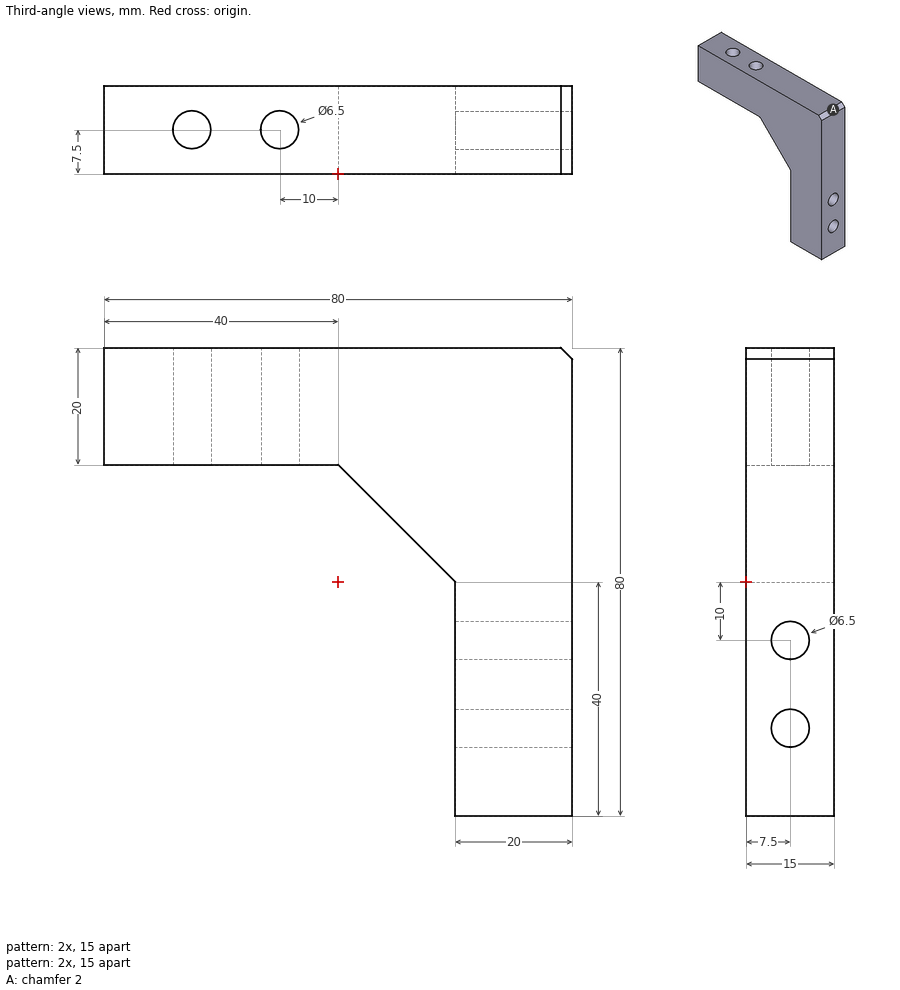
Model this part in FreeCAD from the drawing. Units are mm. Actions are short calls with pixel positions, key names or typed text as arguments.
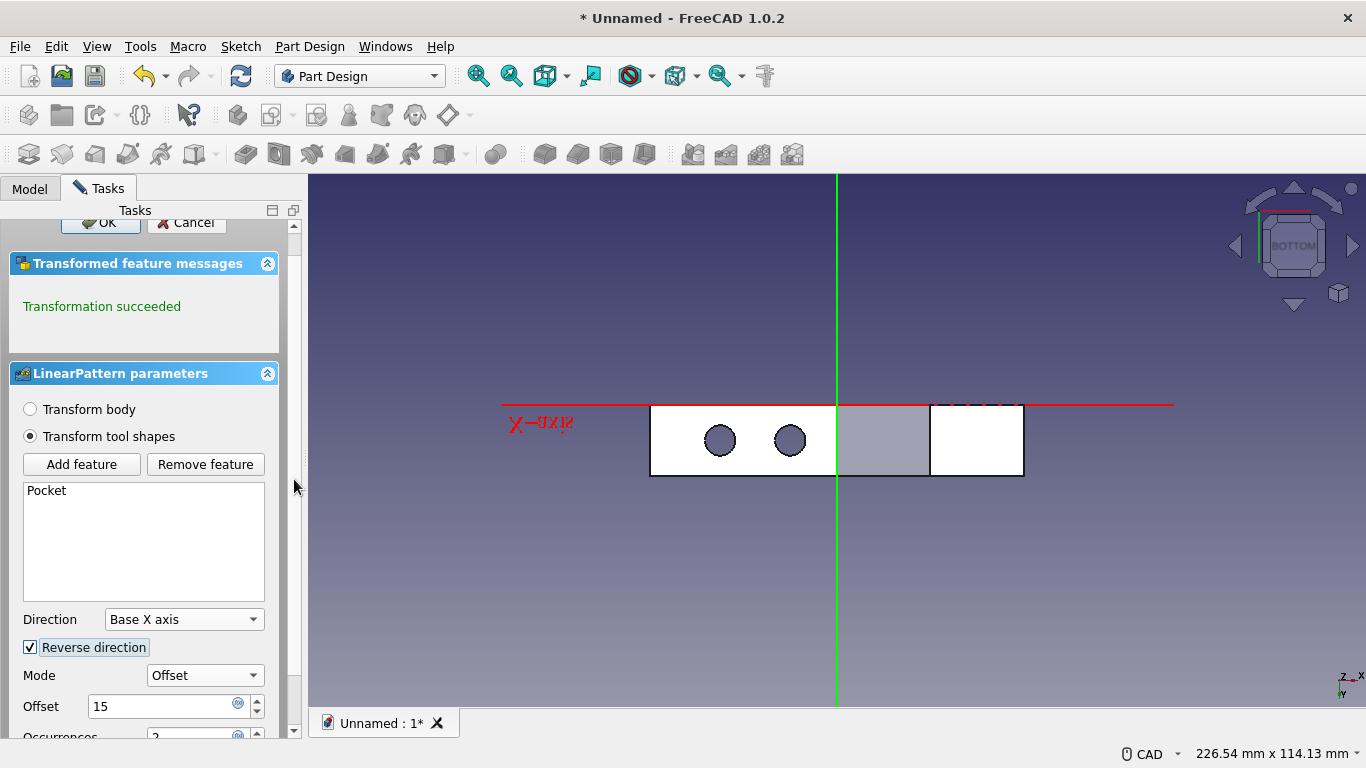
click(101, 249)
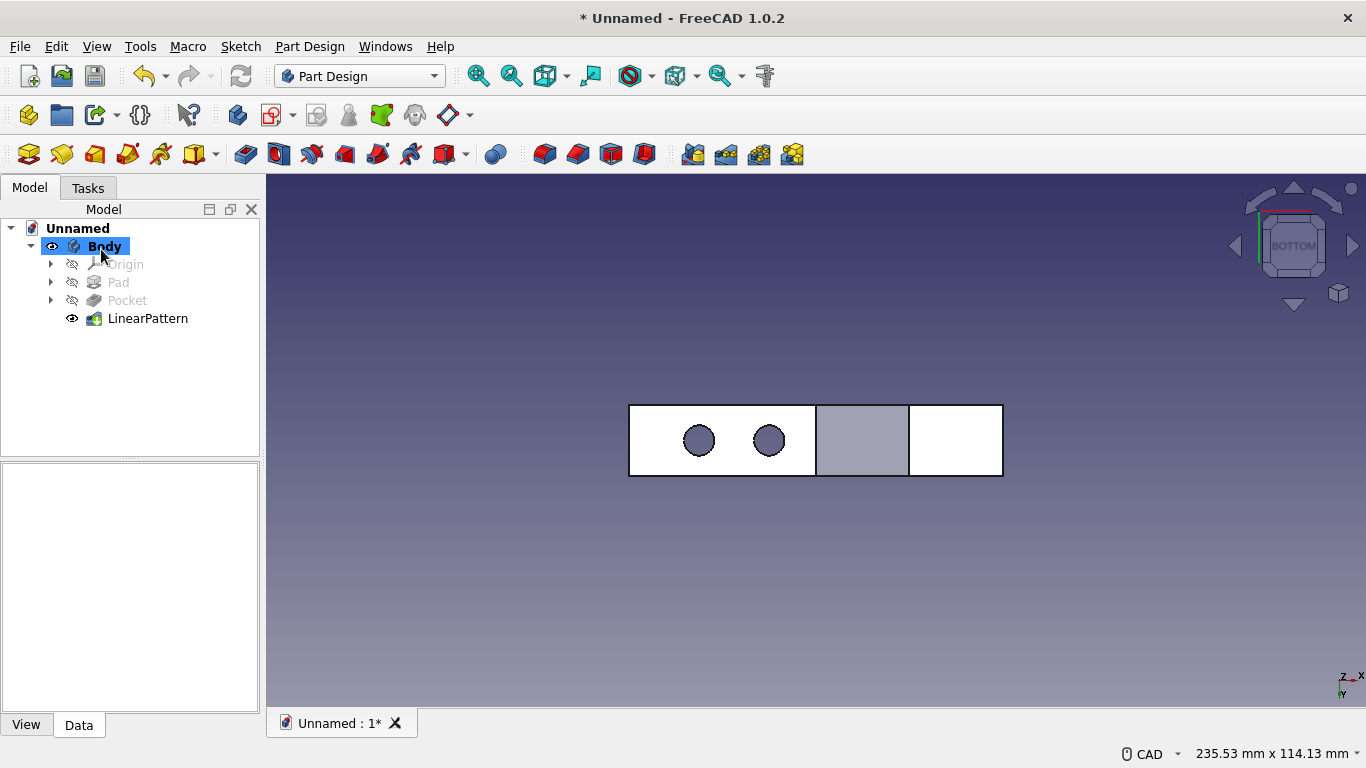
key(v)
key(f)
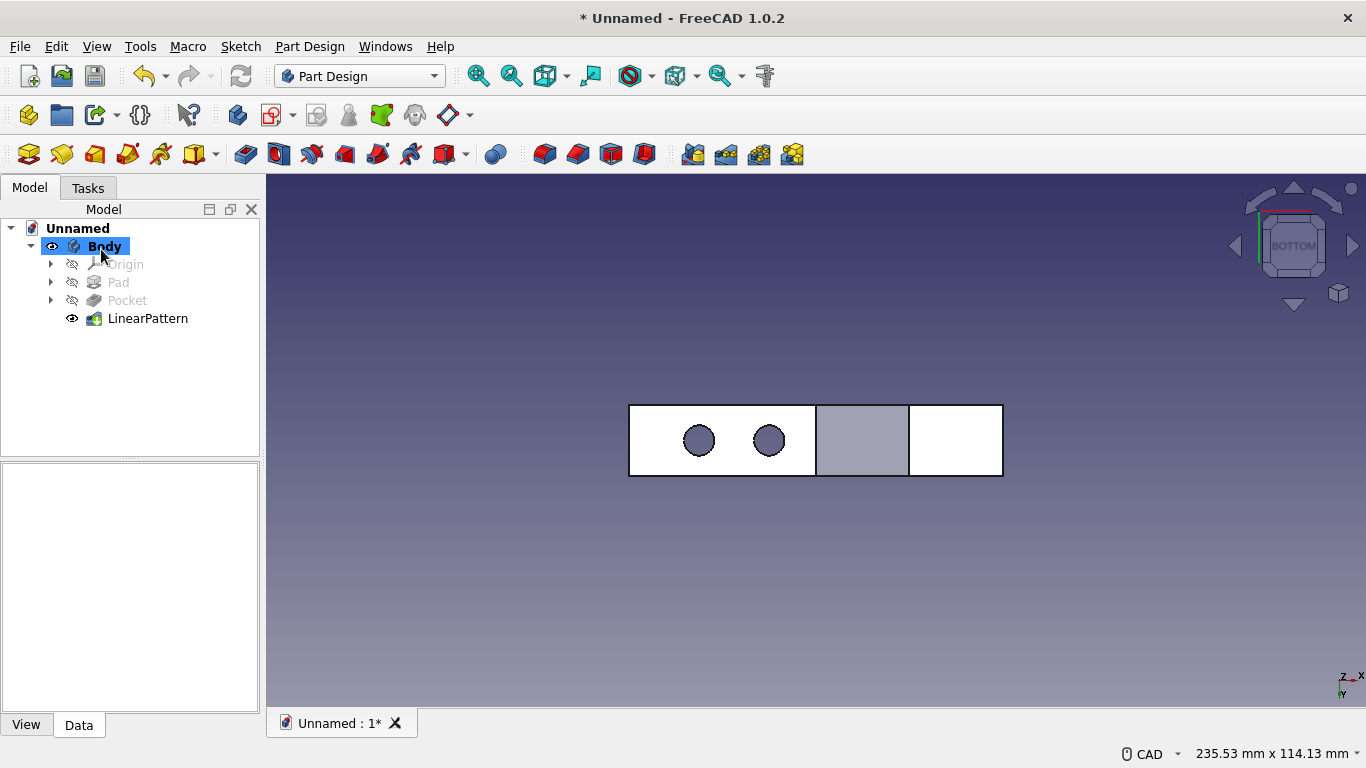
key(0)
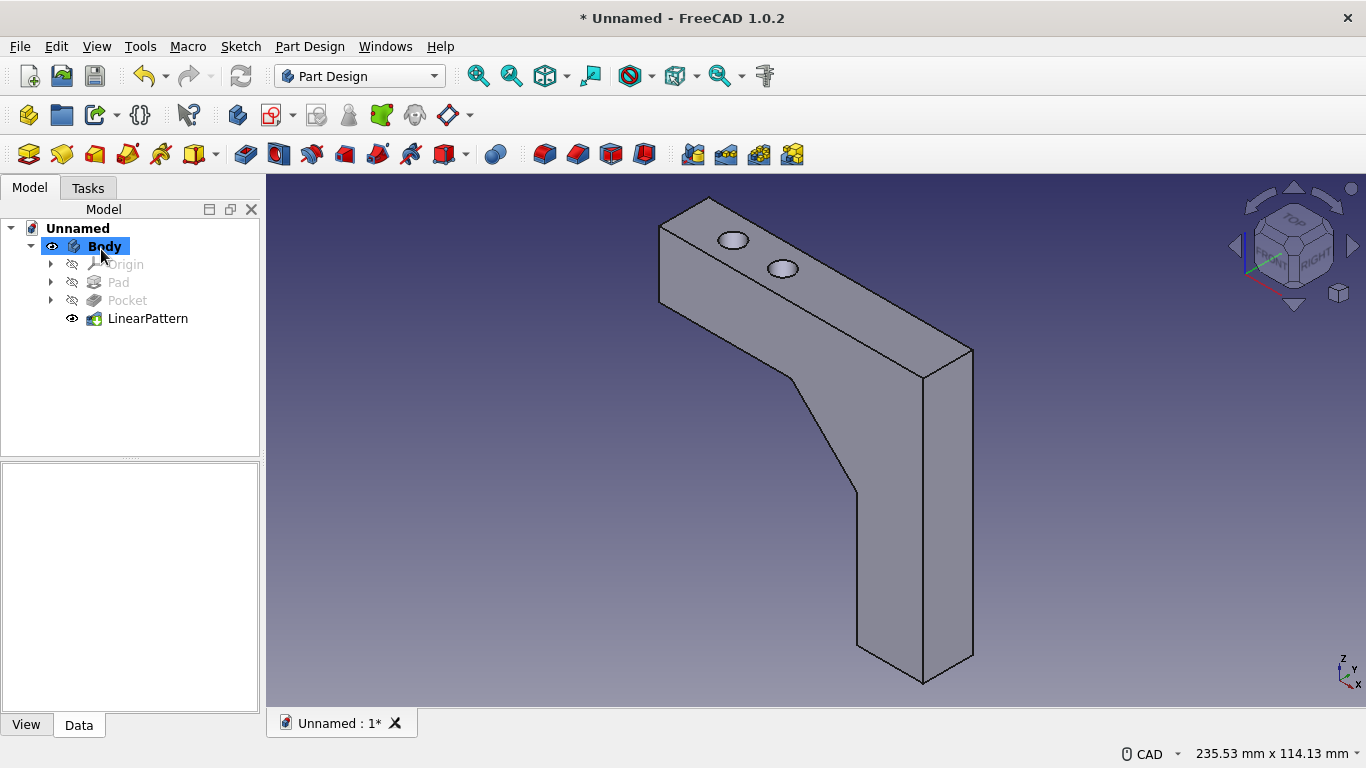
click(948, 516)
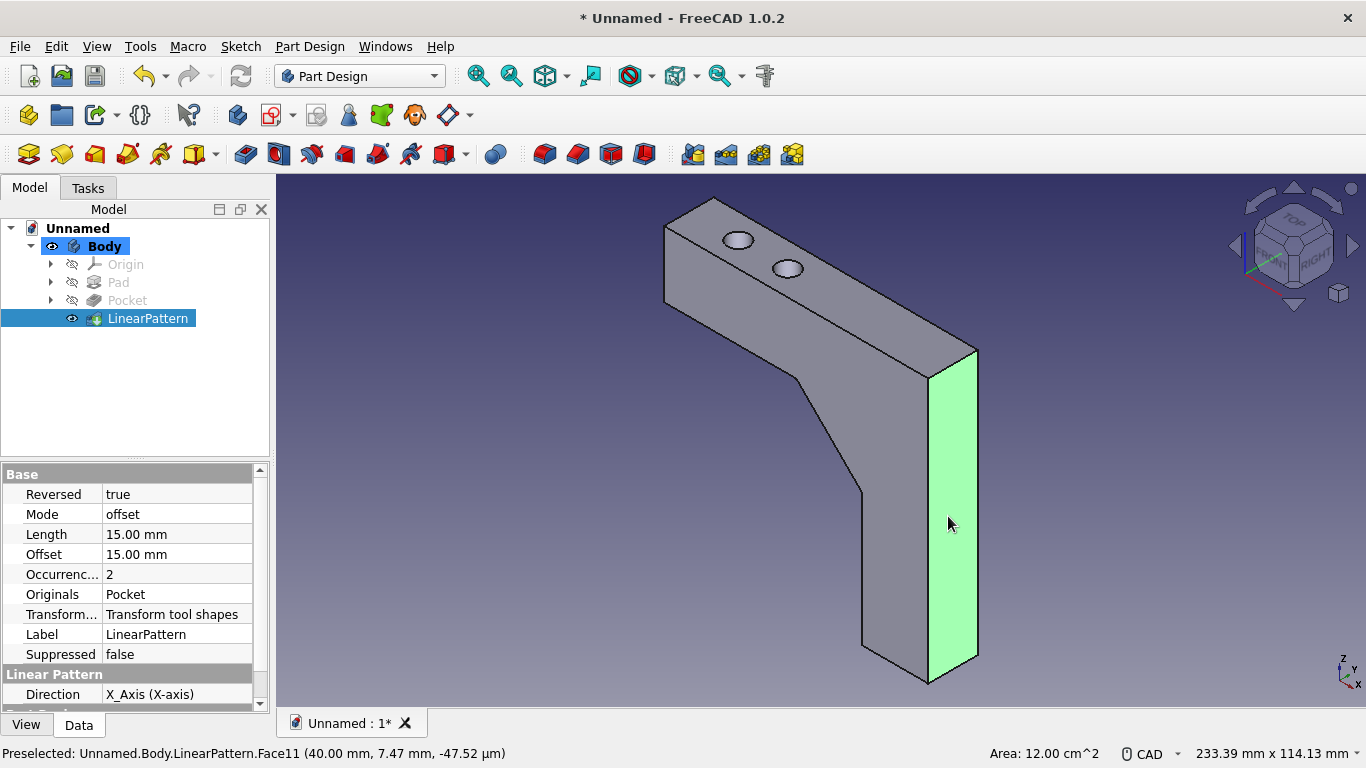
click(270, 116)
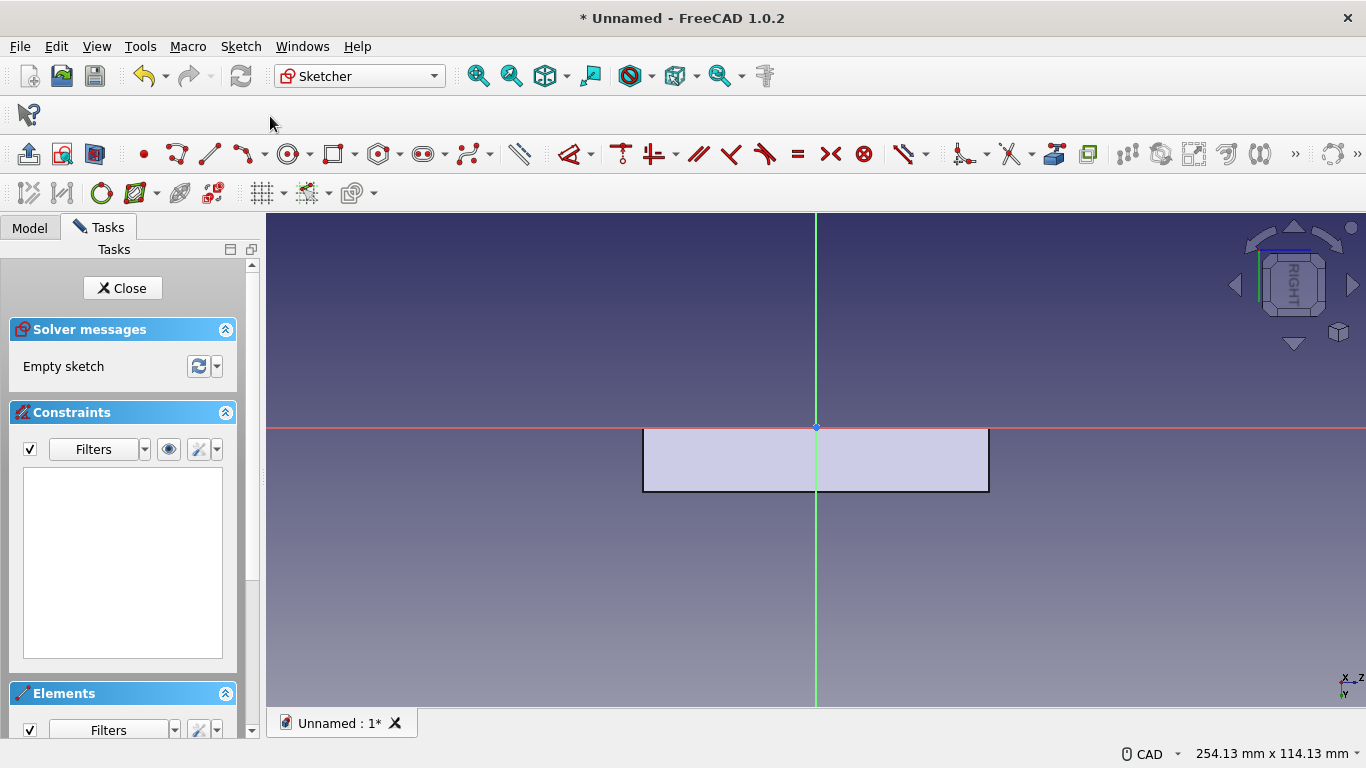
scroll(795, 449, up, 9)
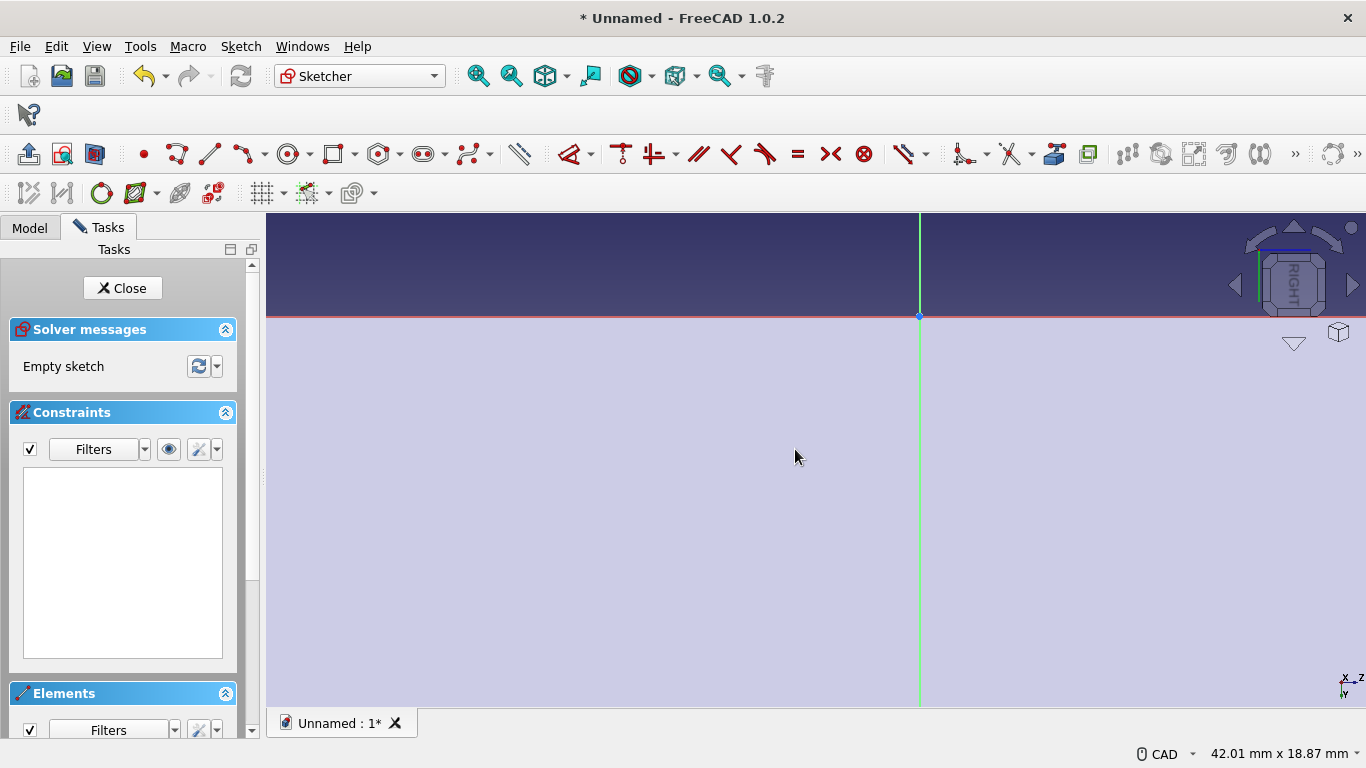
key(g)
key(c)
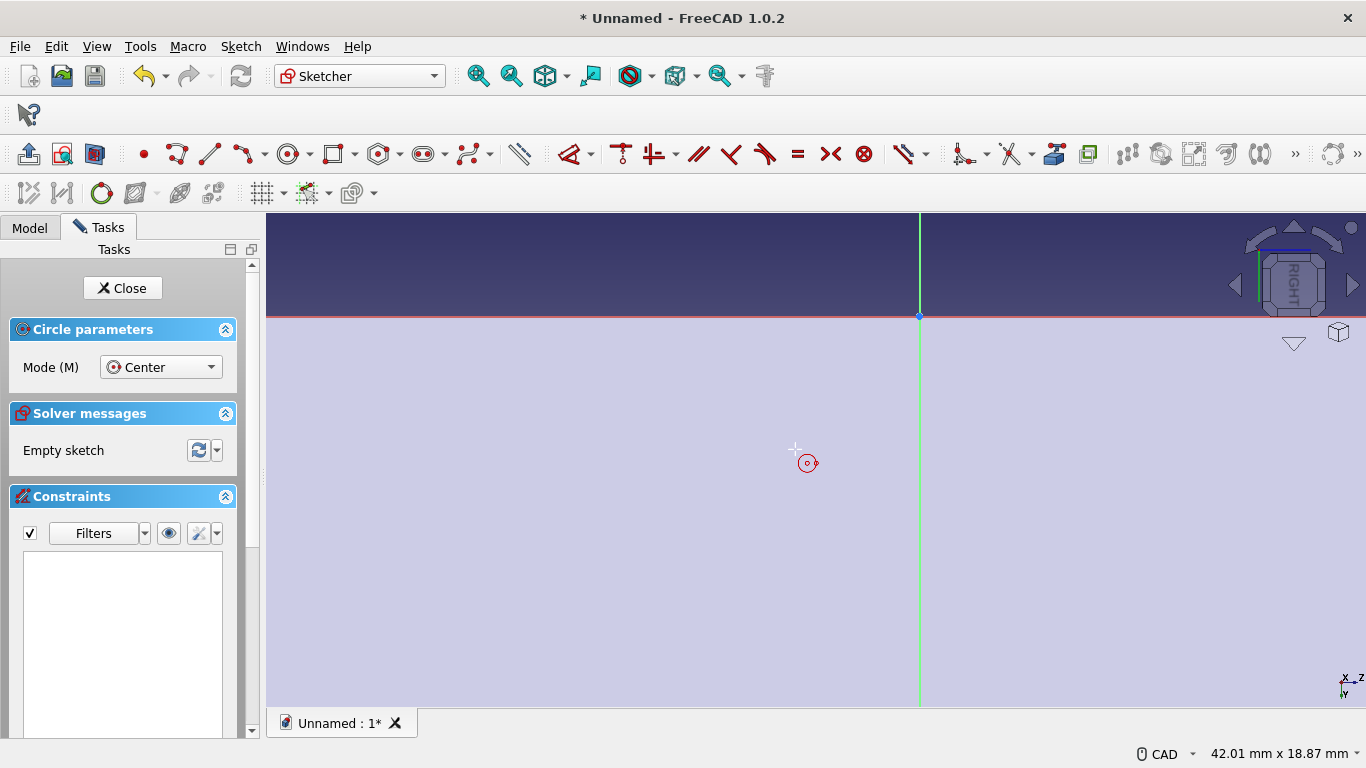
click(658, 513)
move(718, 453)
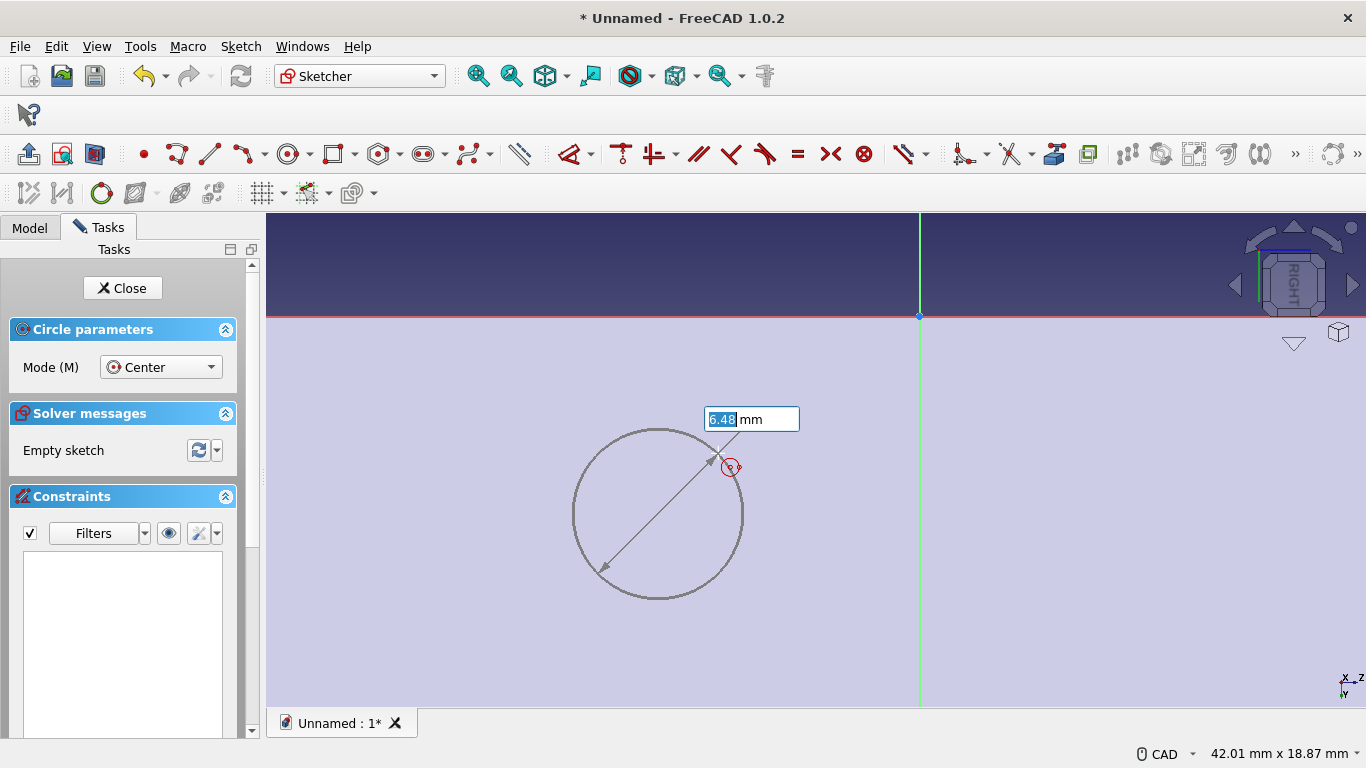
text(6.5)
key(Return)
key(Escape)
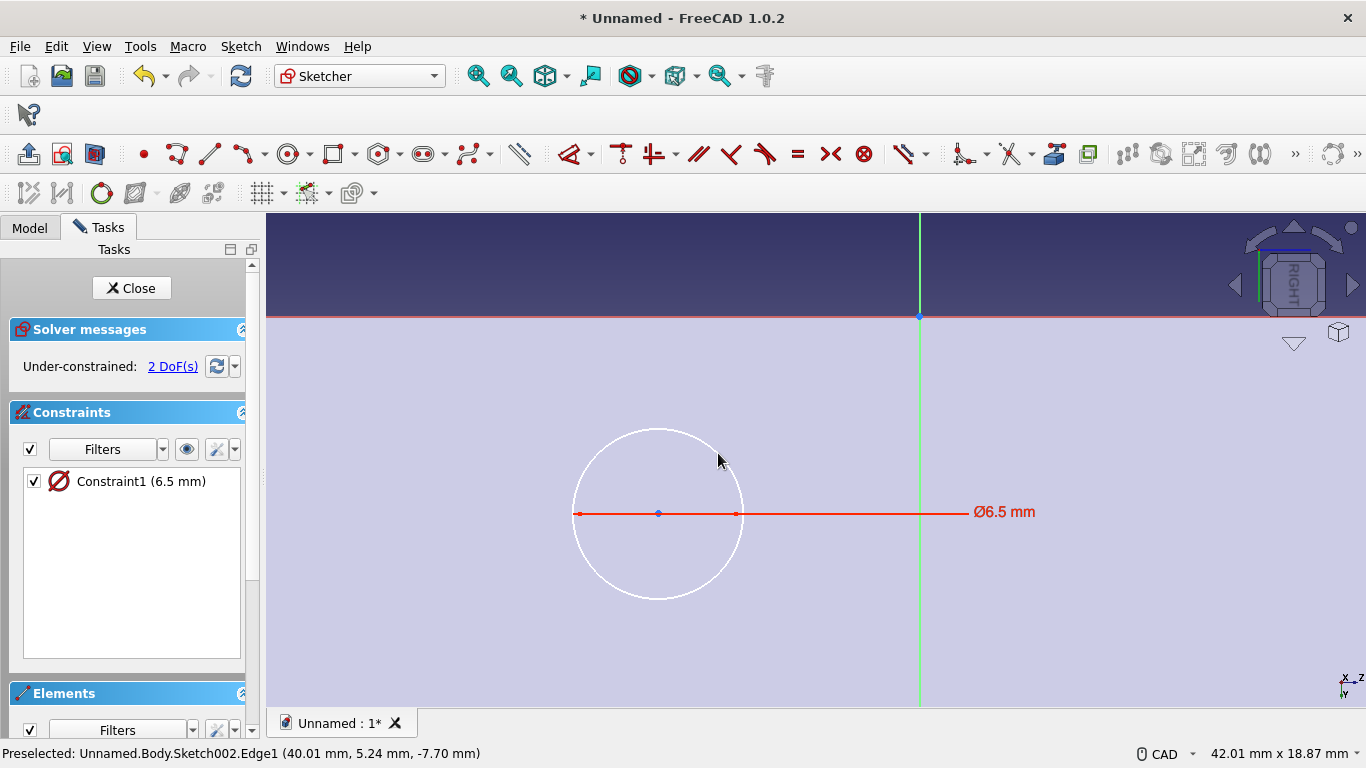
key(d)